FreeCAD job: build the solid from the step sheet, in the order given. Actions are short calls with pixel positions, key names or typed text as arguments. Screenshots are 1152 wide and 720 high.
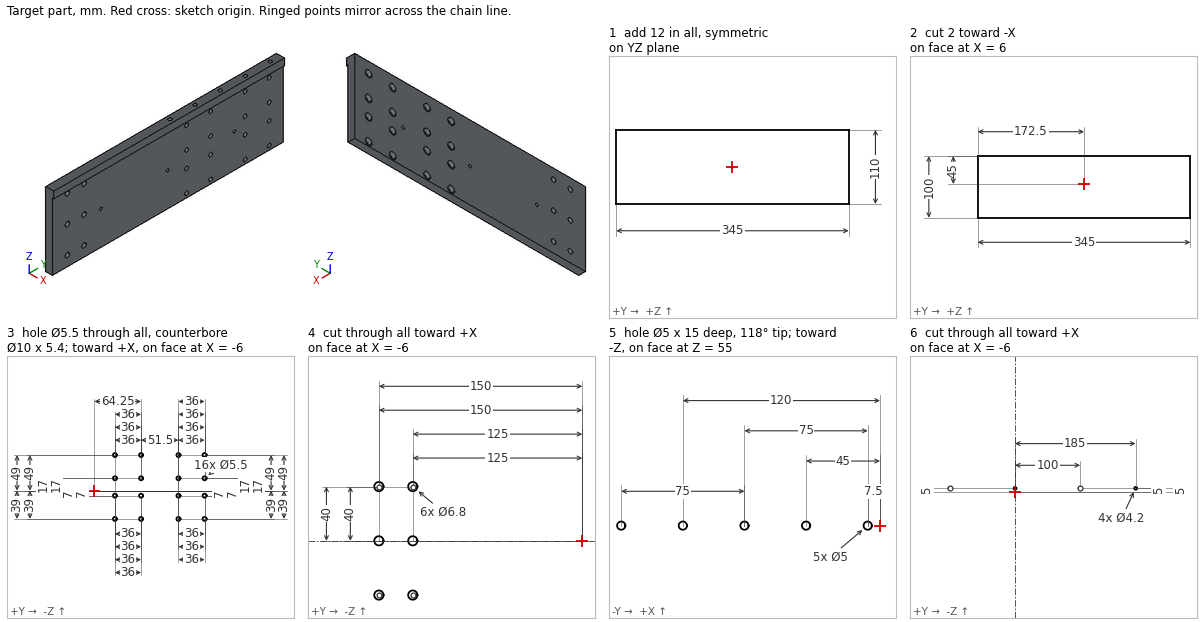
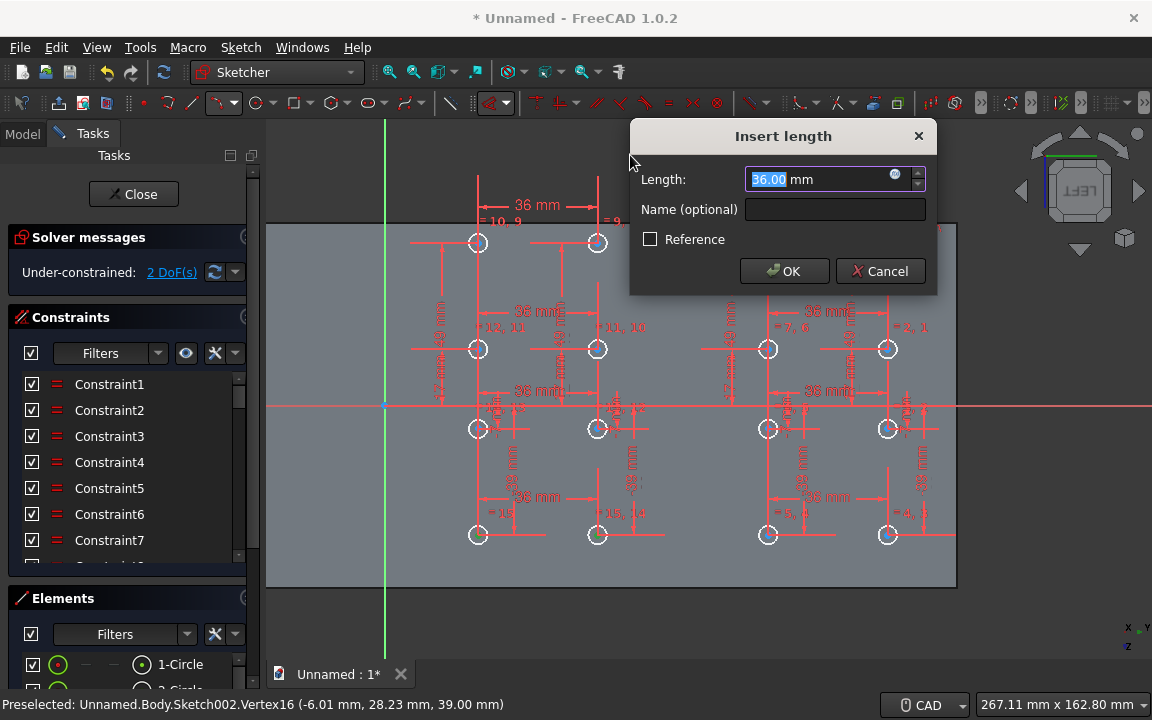
text(36)
key(Return)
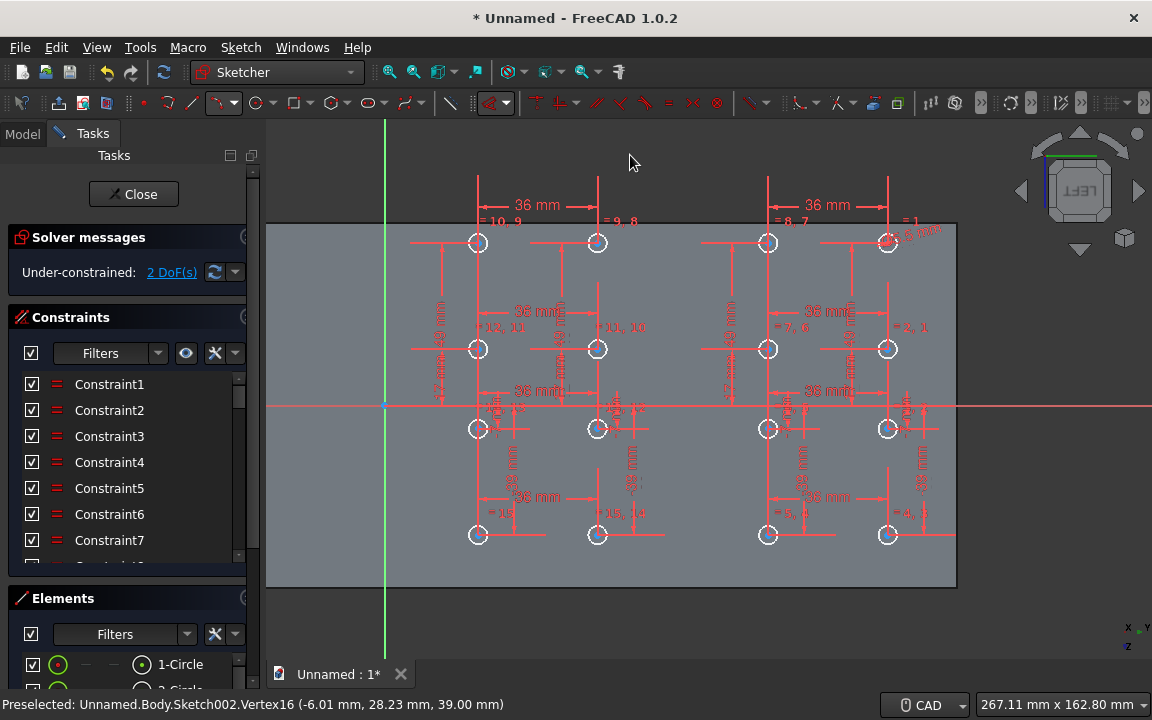
click(598, 243)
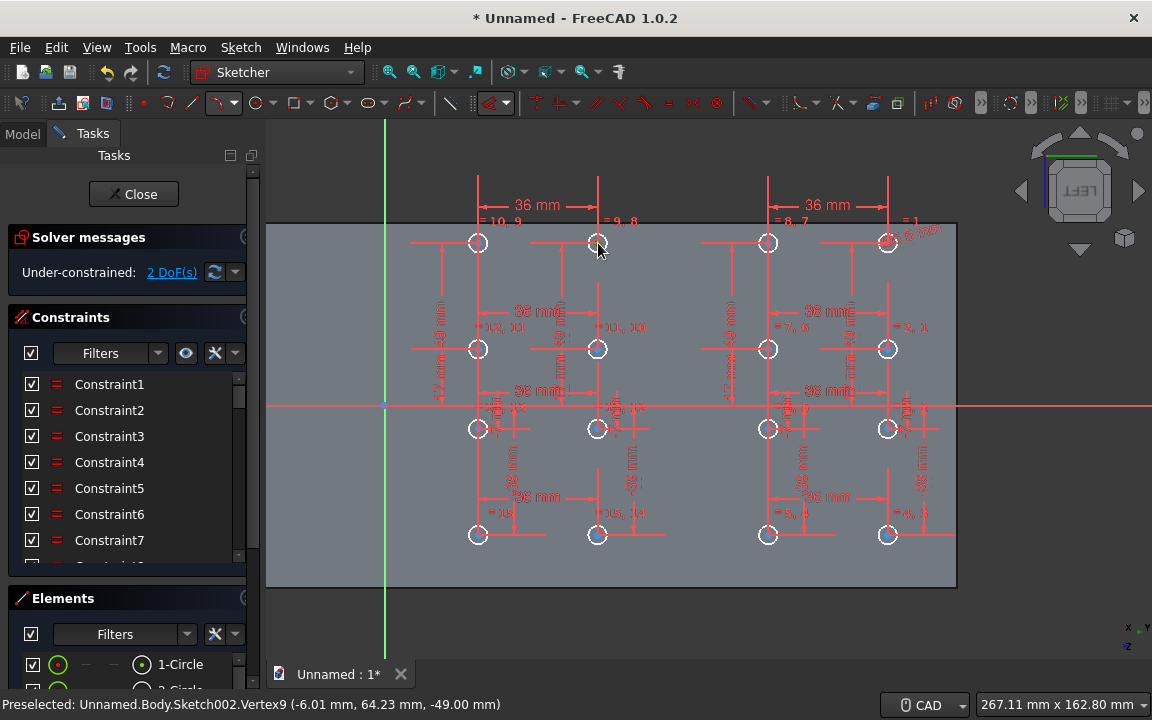
click(508, 104)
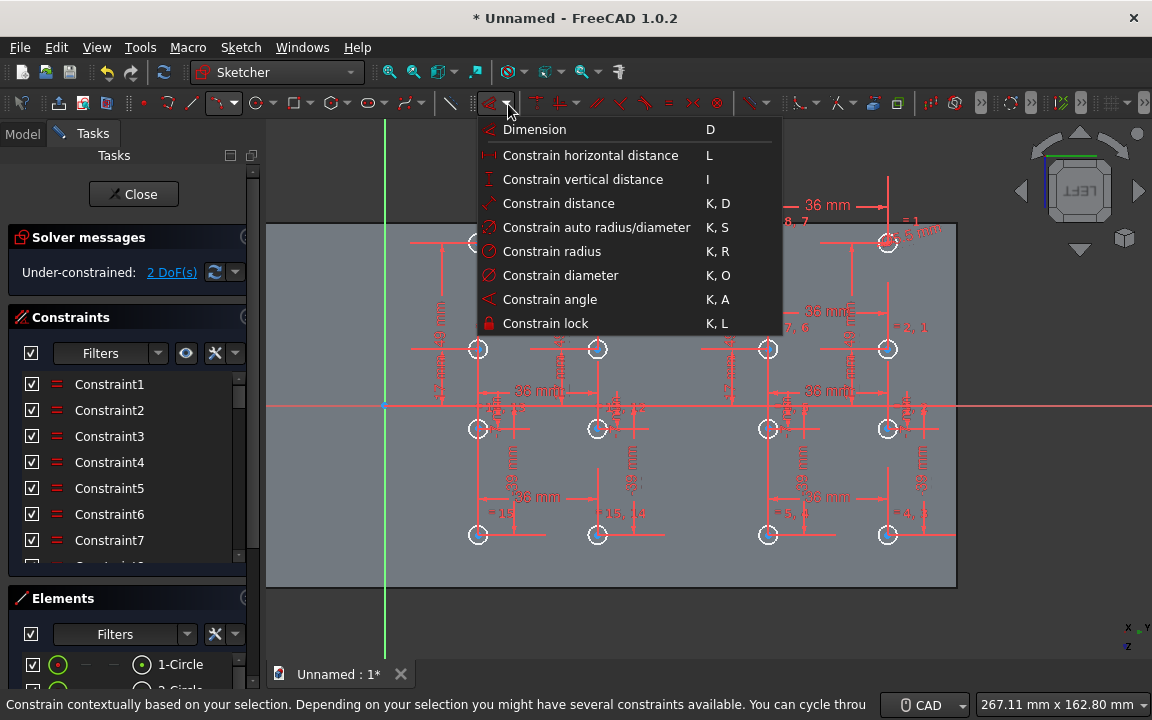
click(630, 155)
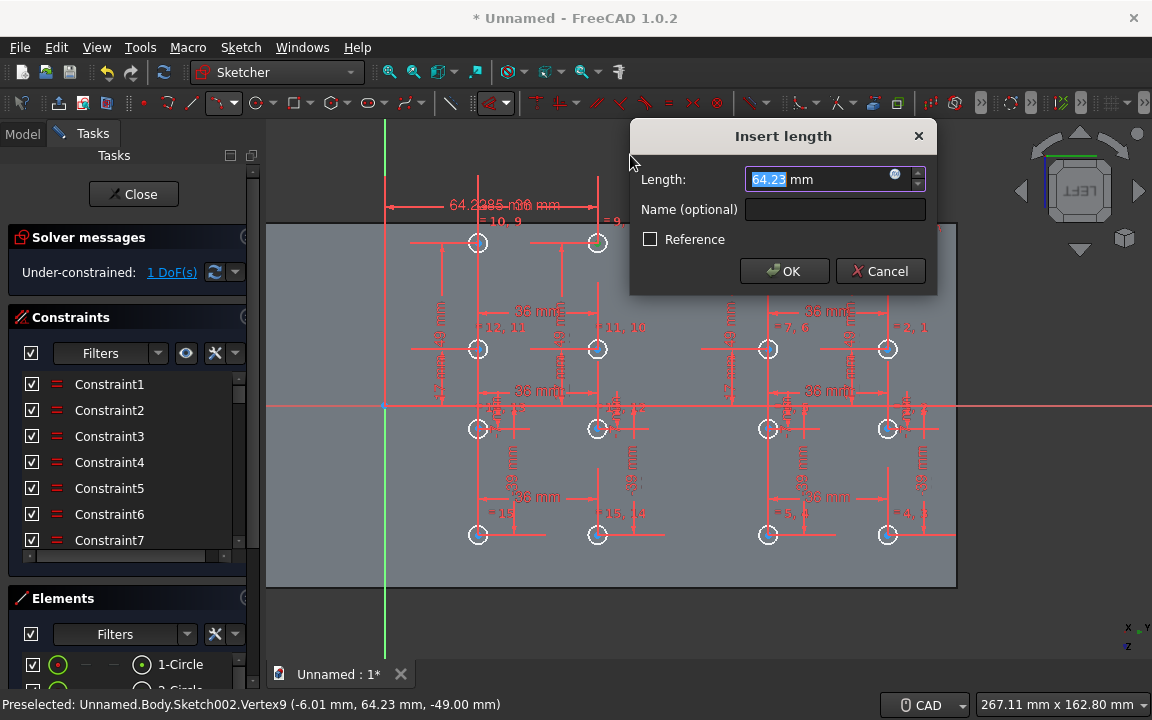
text(64.25)
key(Return)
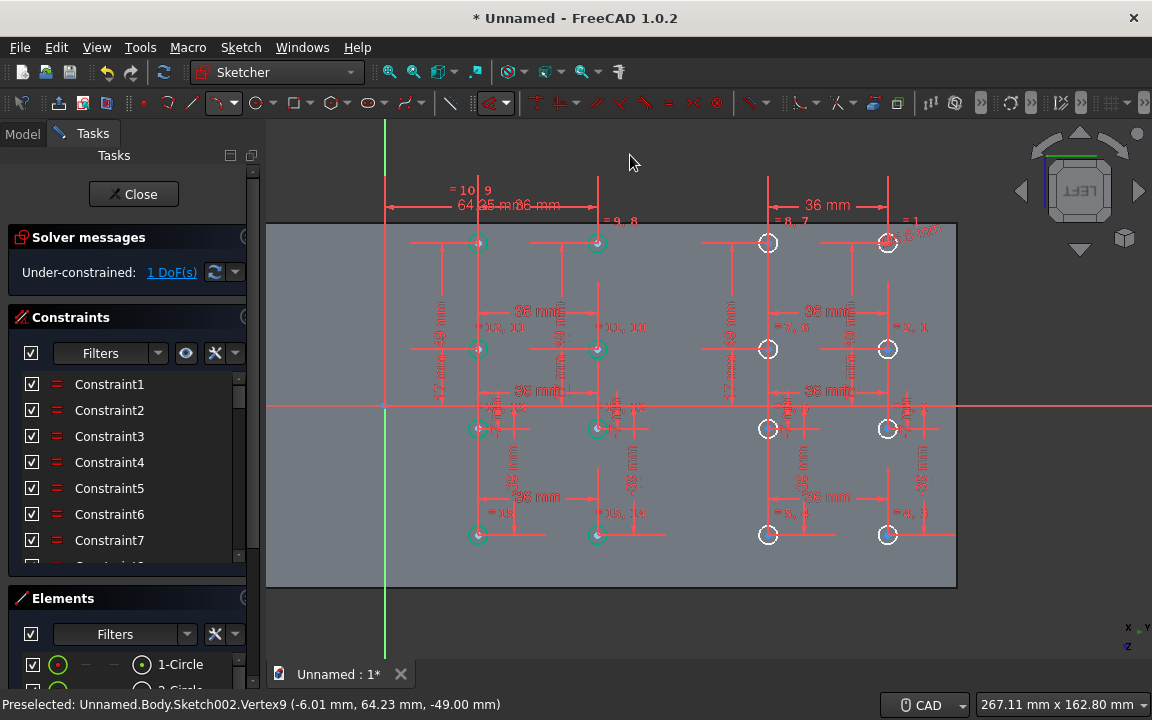
click(768, 243)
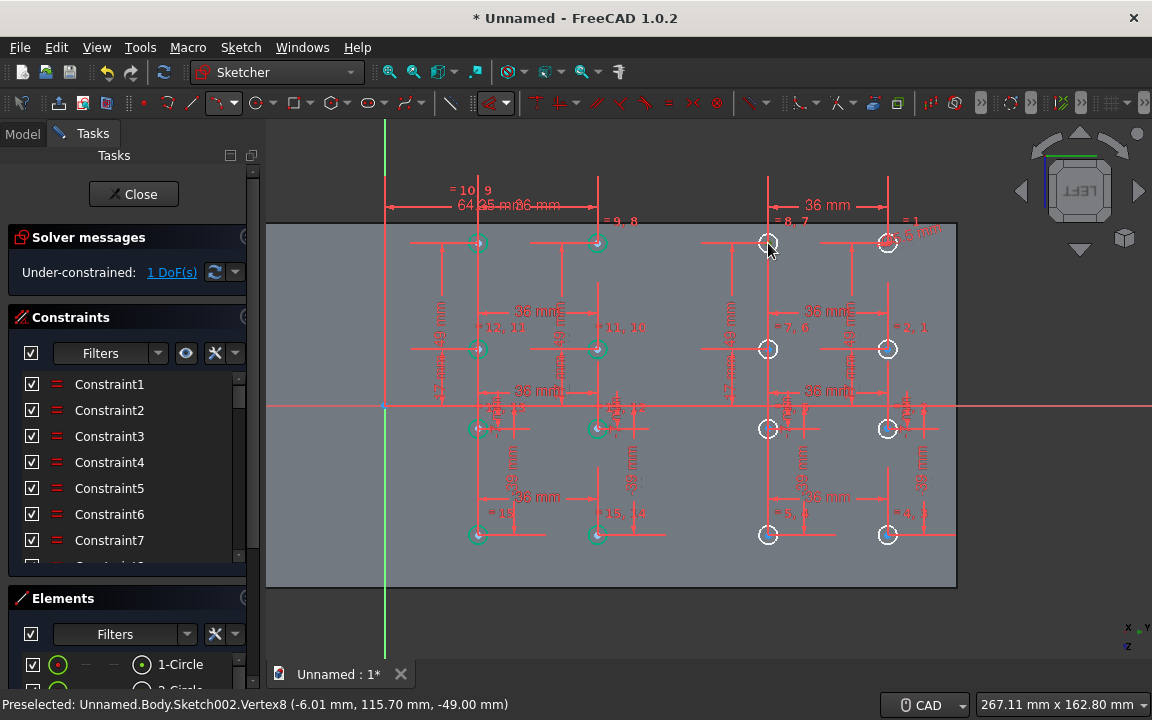
click(598, 243)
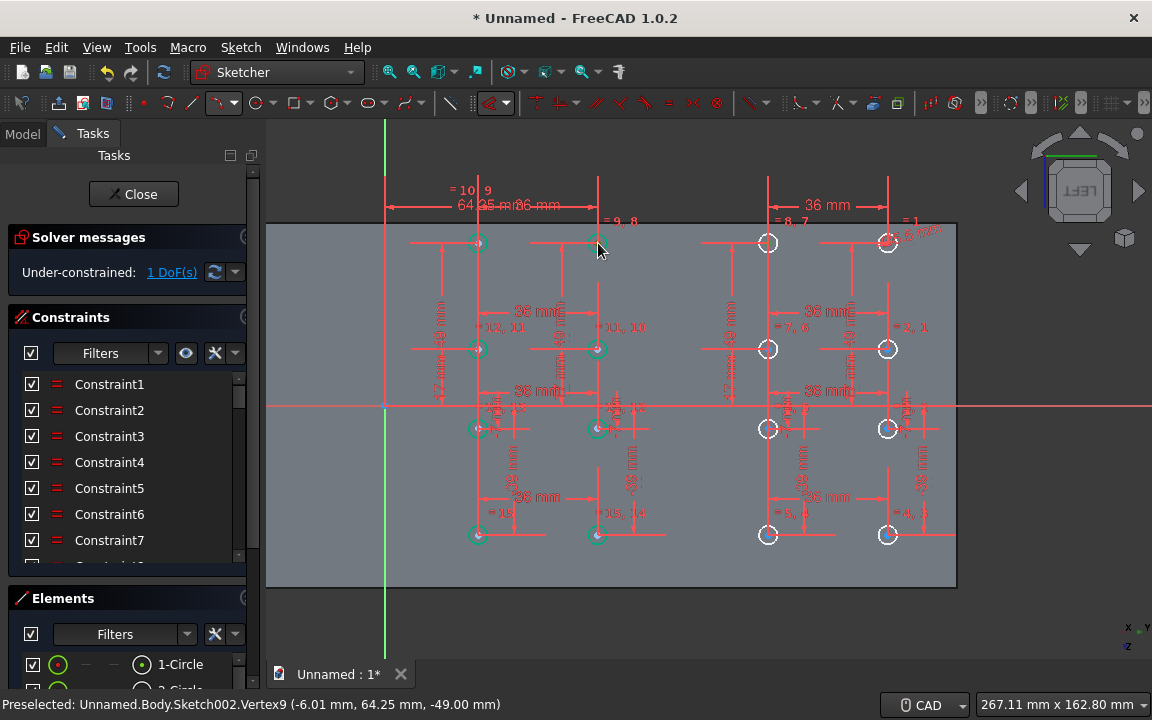
click(508, 104)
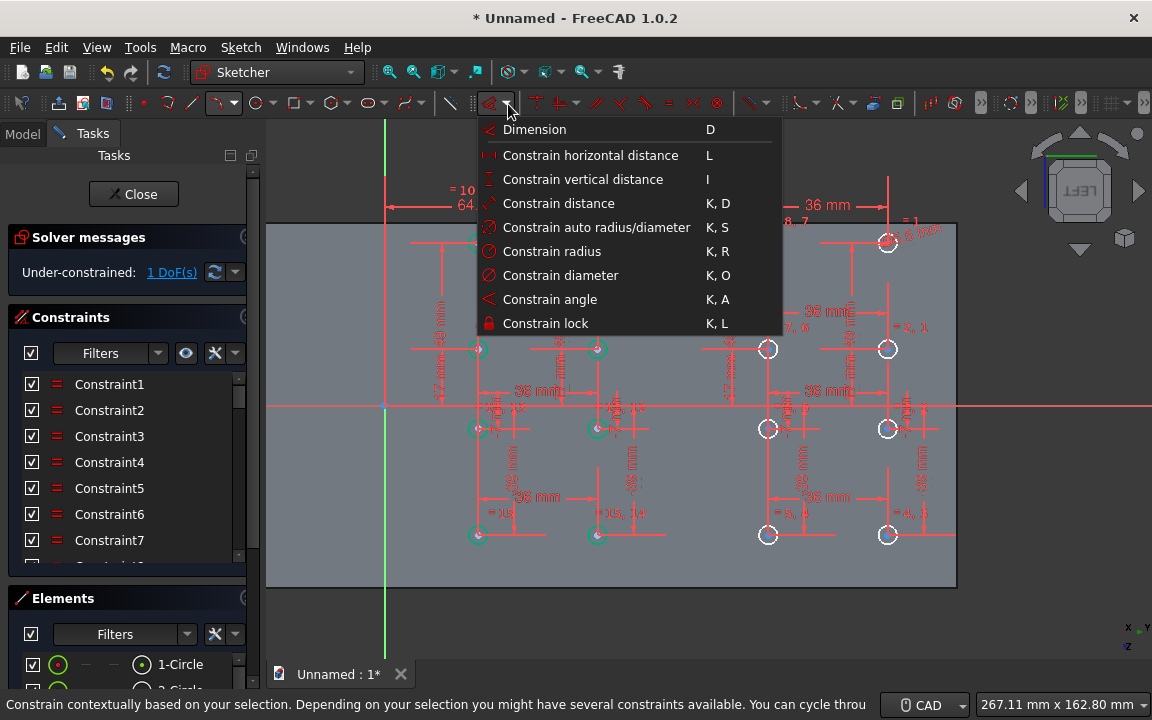
click(630, 155)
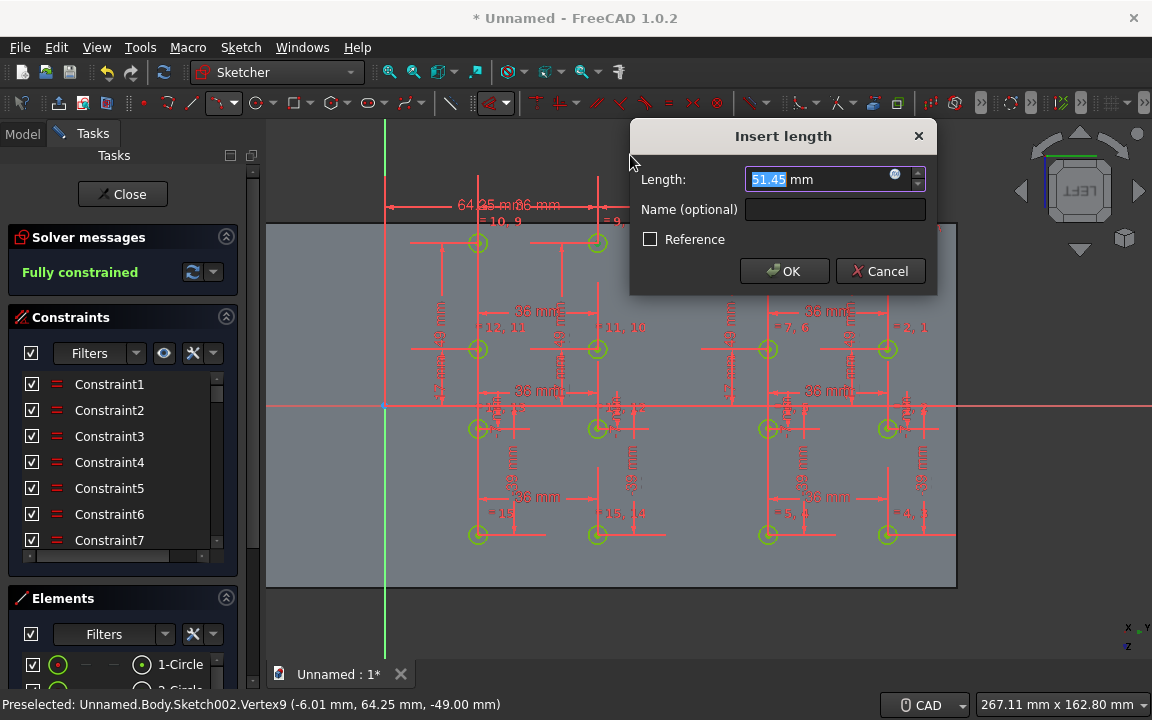
text(51.5)
key(Return)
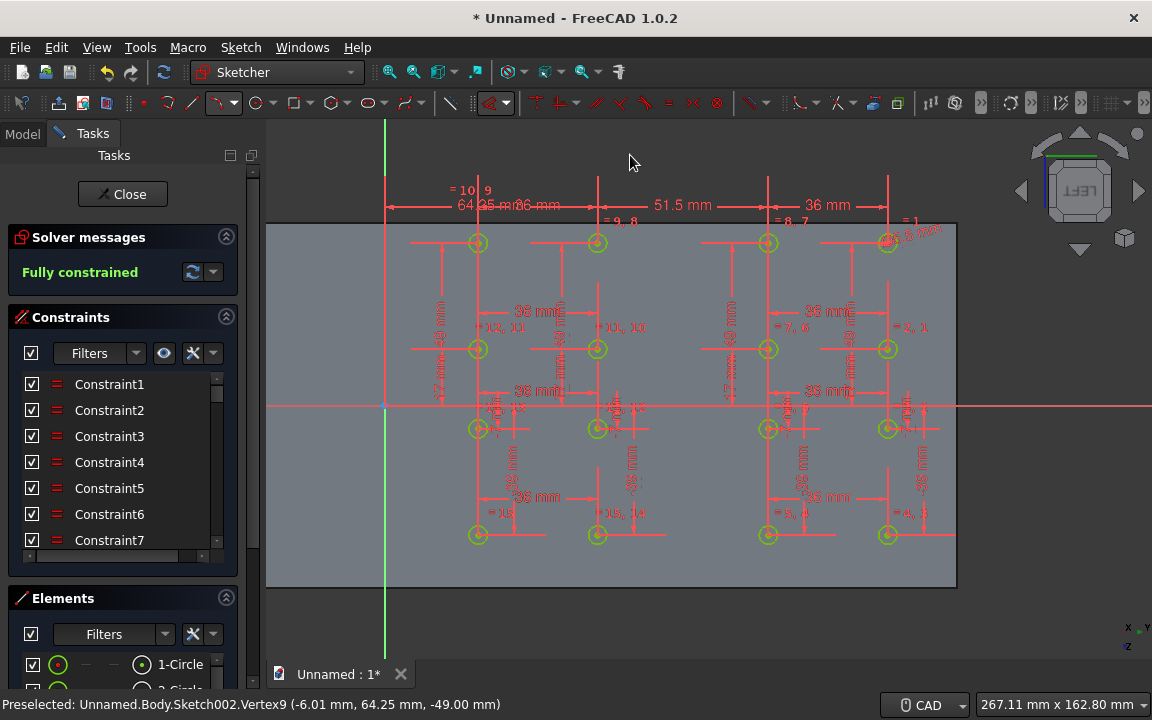
click(123, 194)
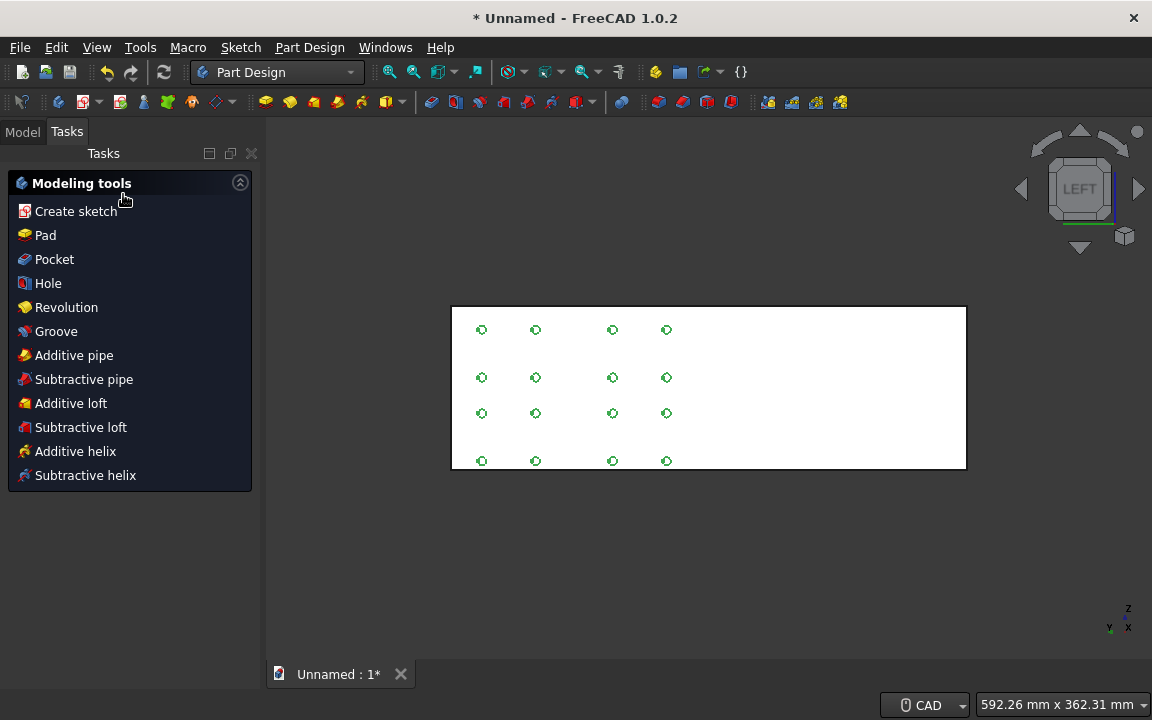
click(456, 102)